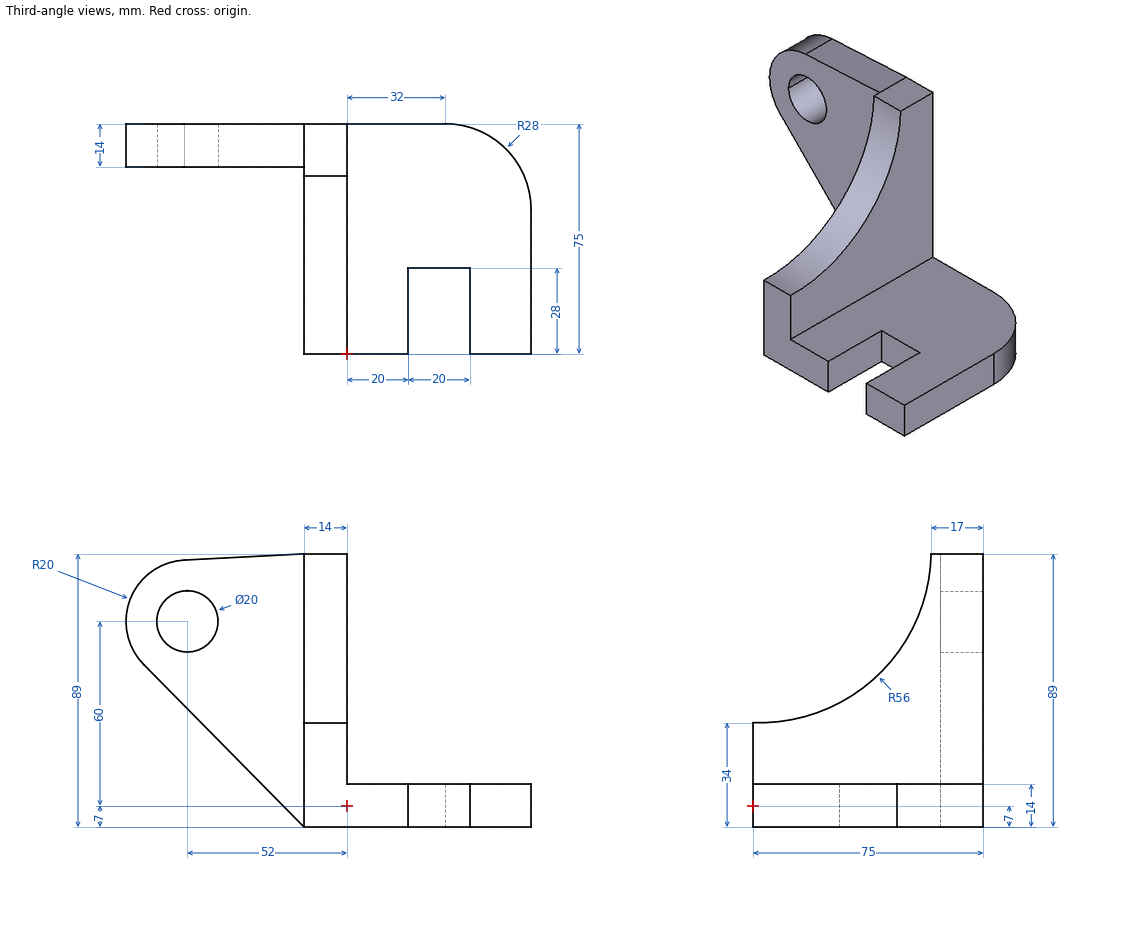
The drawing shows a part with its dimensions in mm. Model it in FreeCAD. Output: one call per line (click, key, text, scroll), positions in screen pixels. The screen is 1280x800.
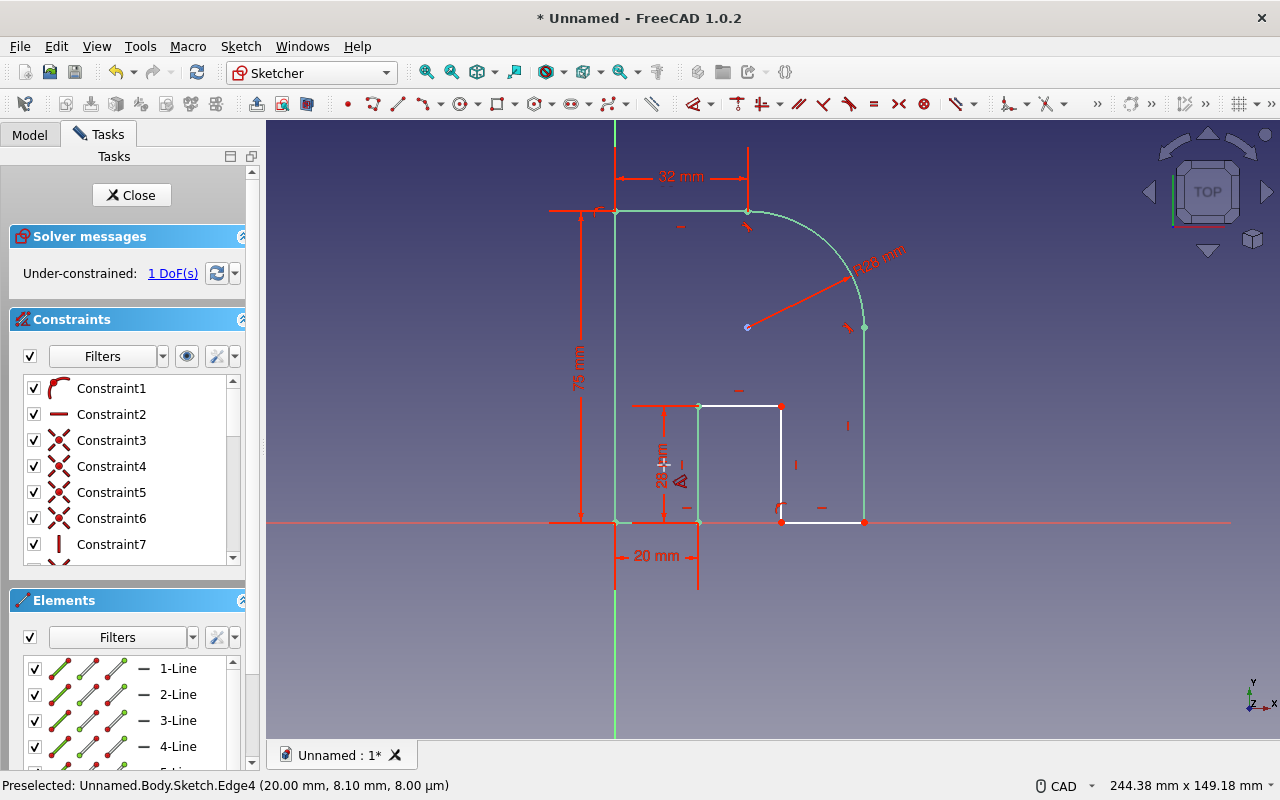
click(723, 406)
click(740, 440)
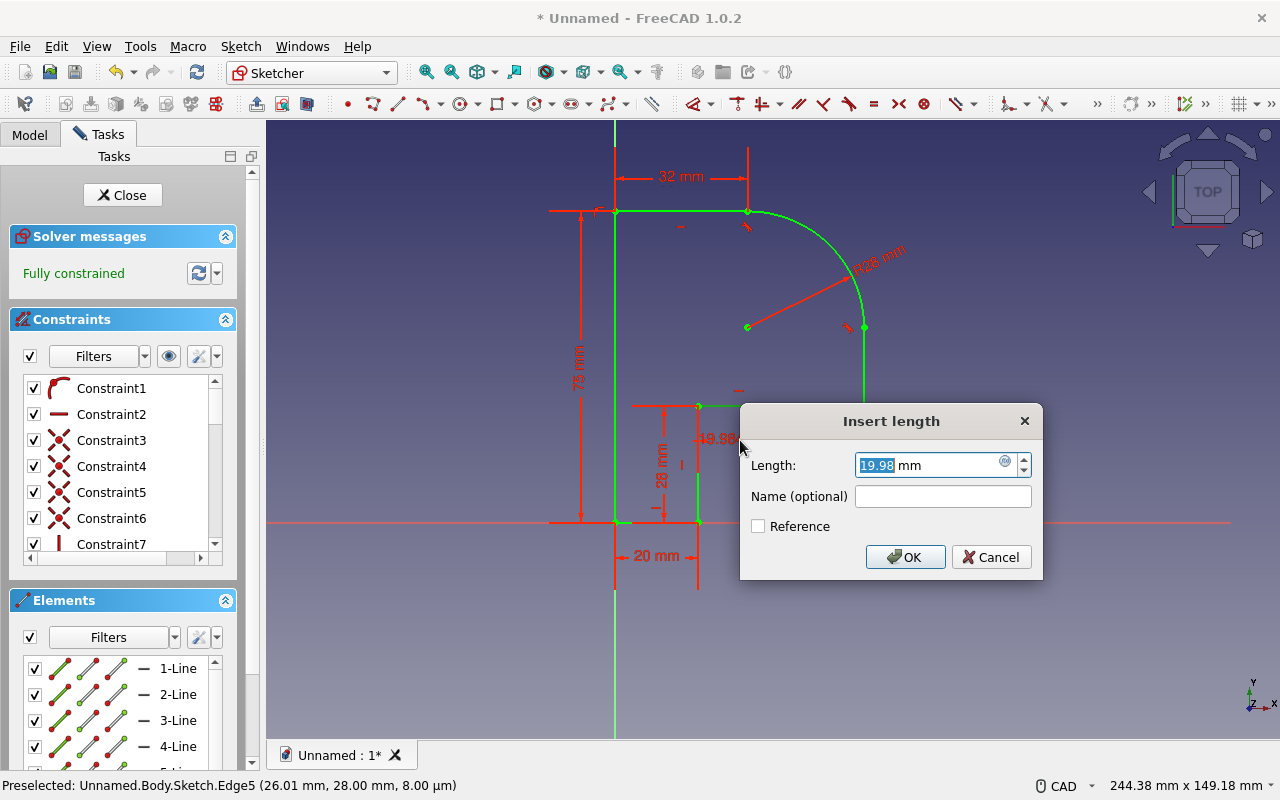
text(20)
key(Return)
key(Escape)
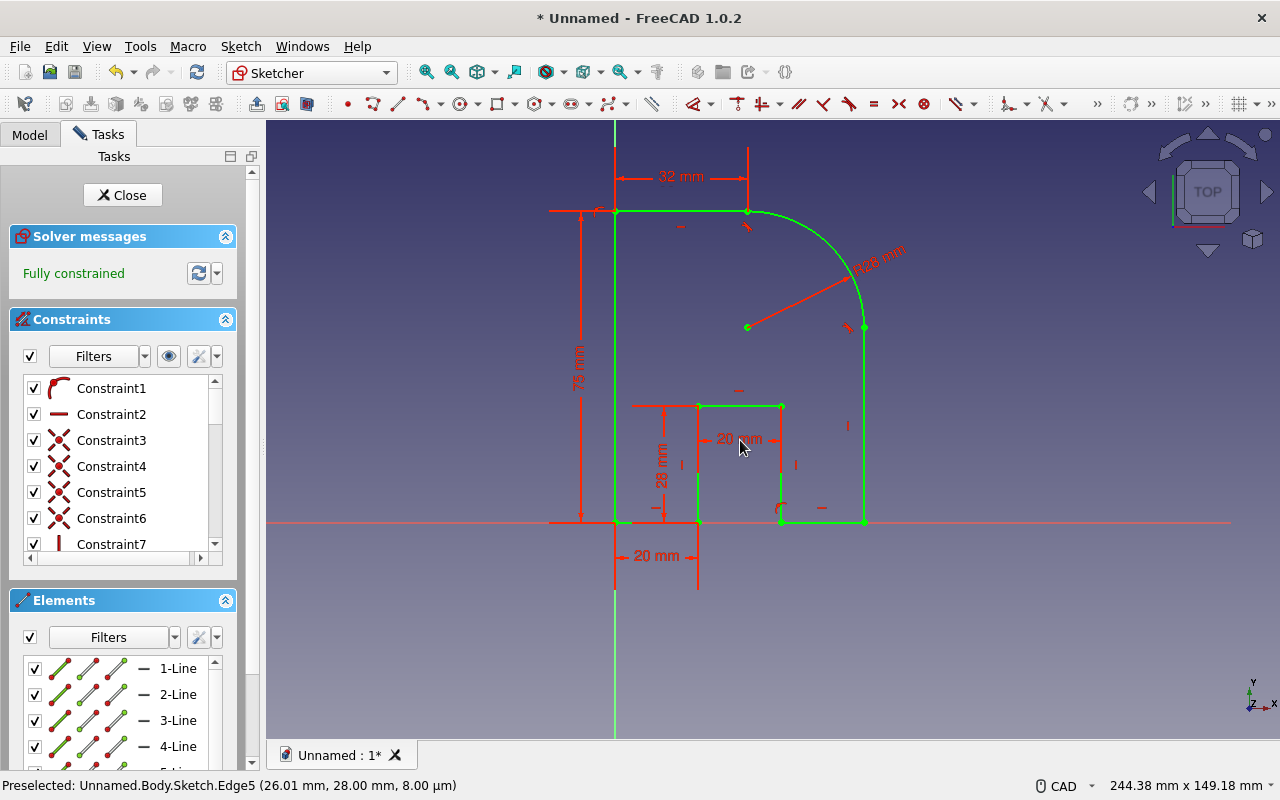
click(123, 195)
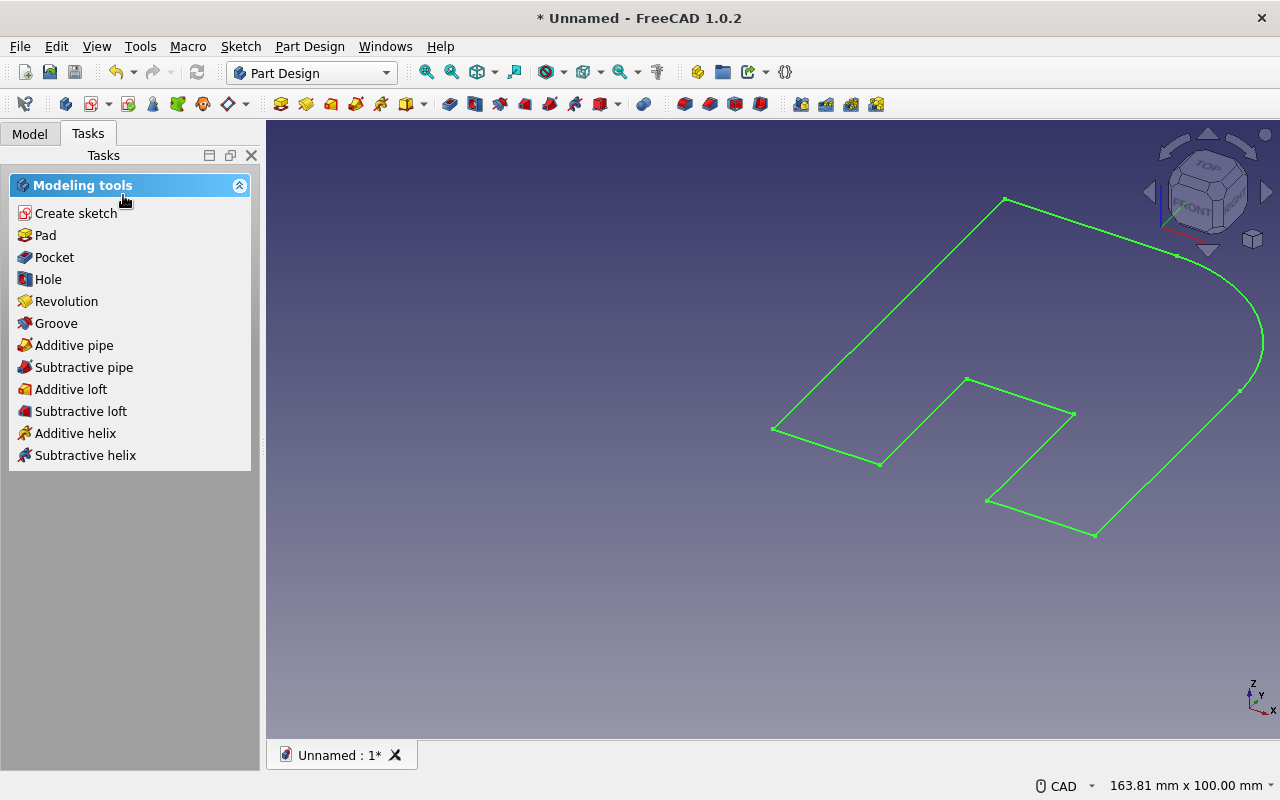
click(281, 104)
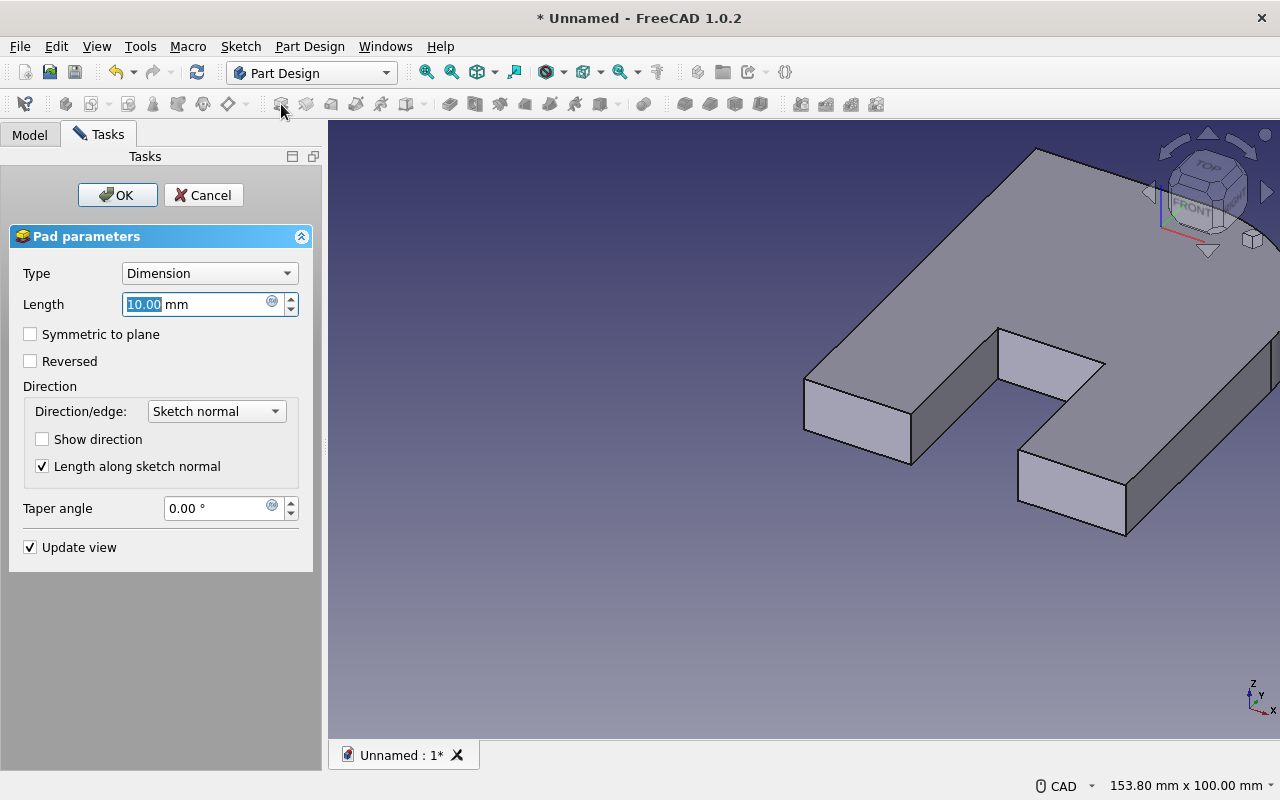
text(14)
key(Tab)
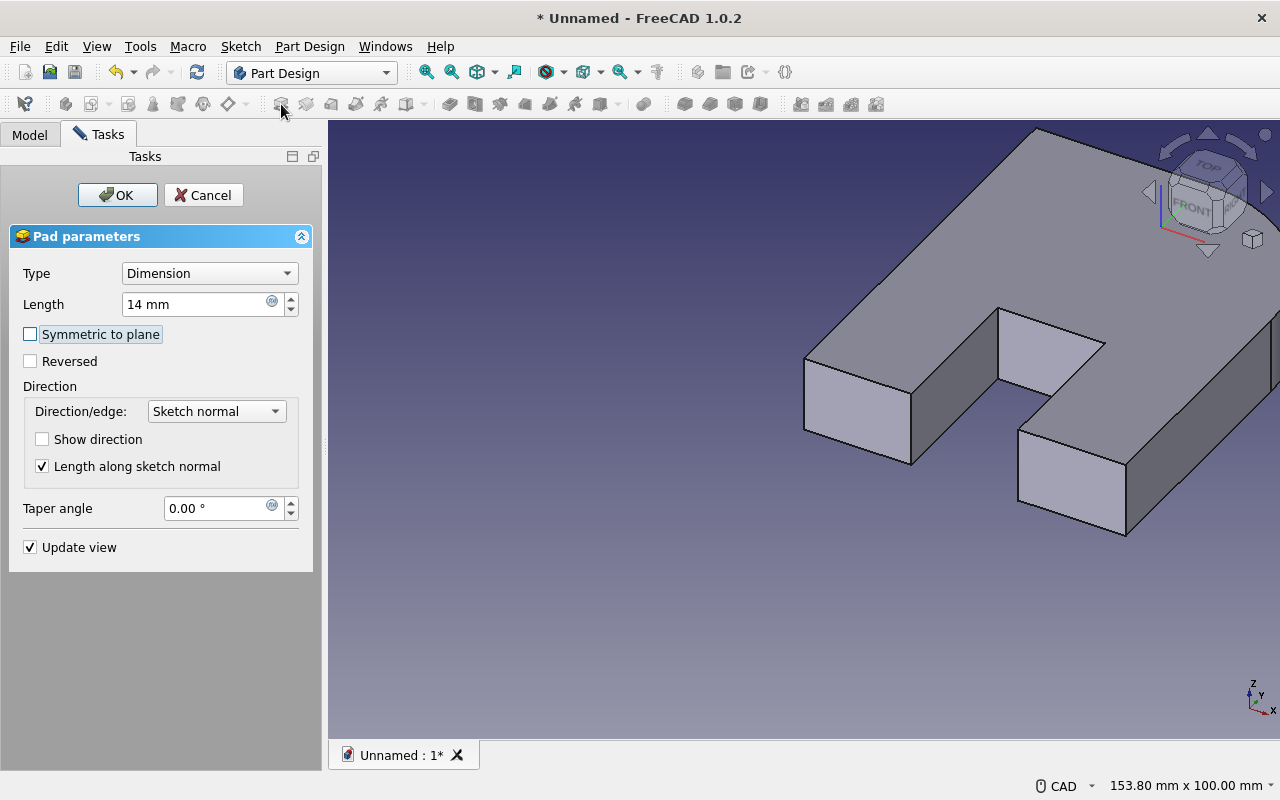
click(31, 334)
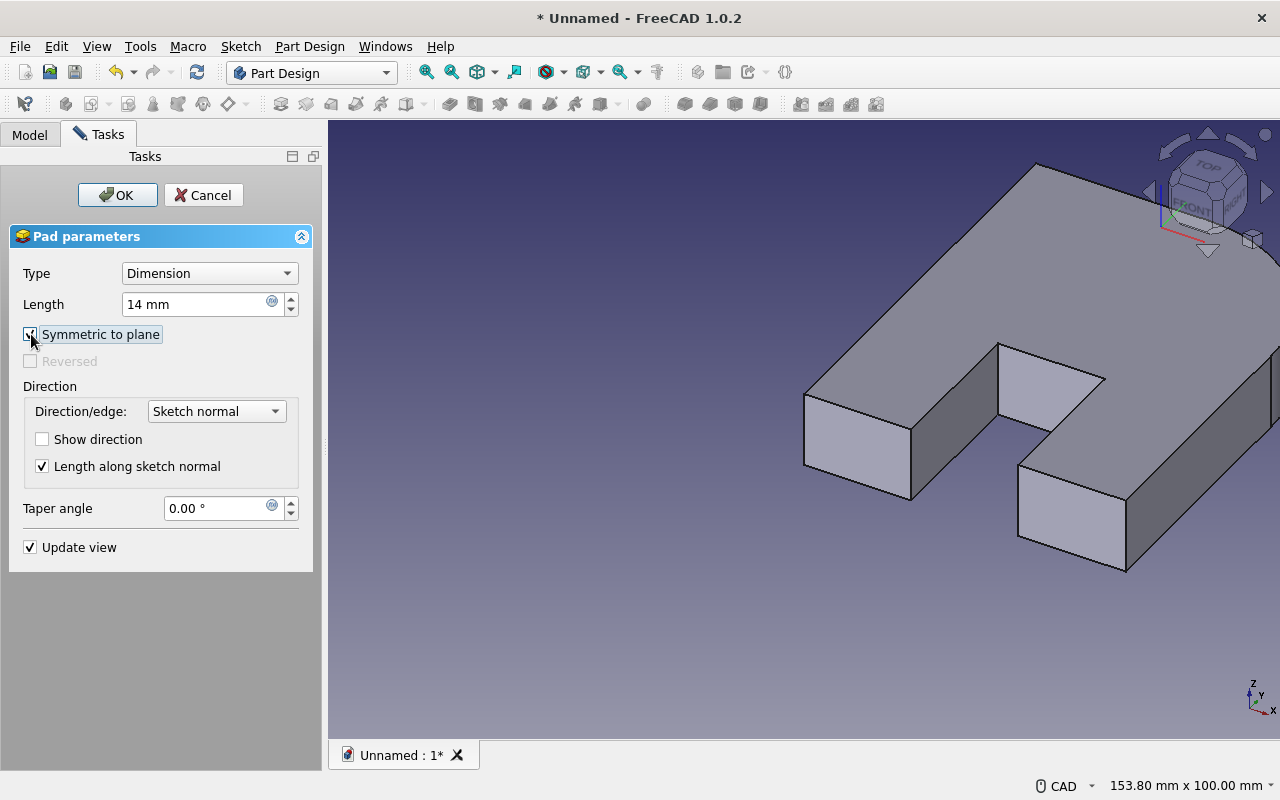
click(118, 195)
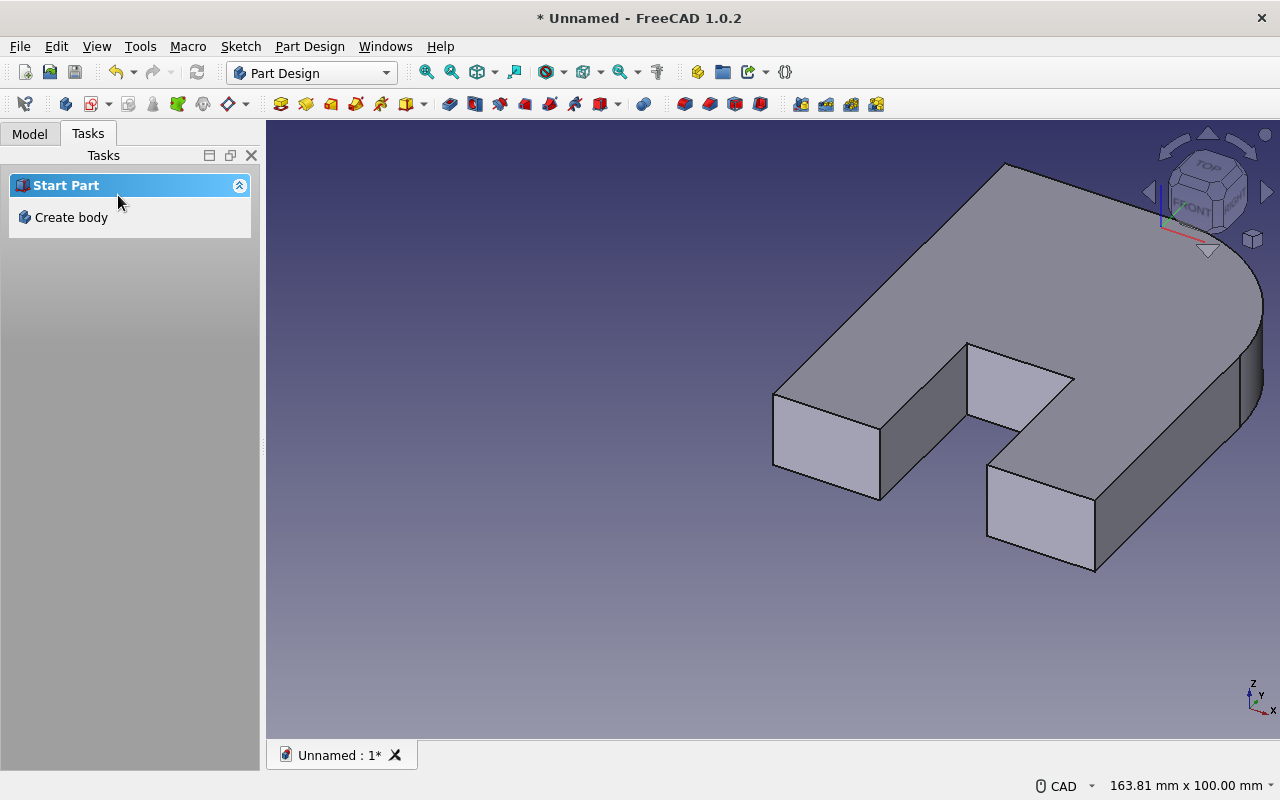
click(427, 72)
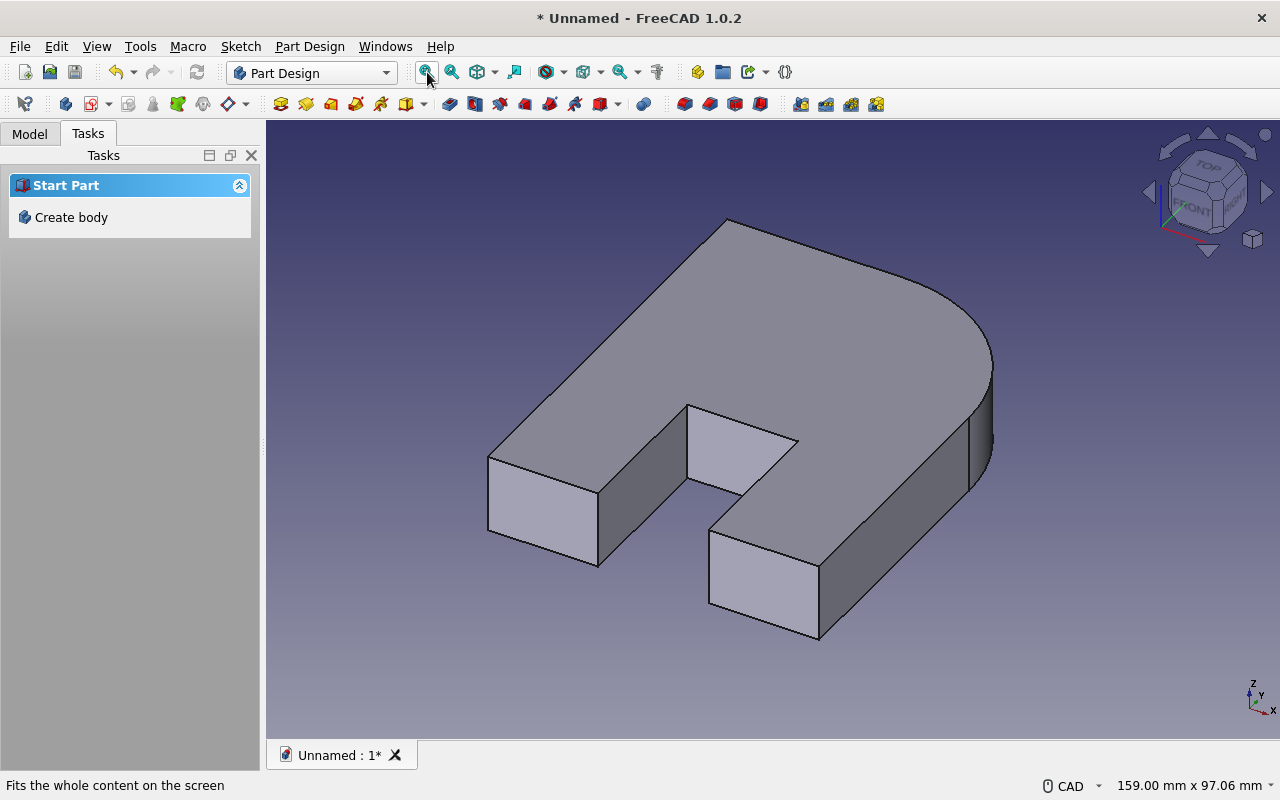
key(6)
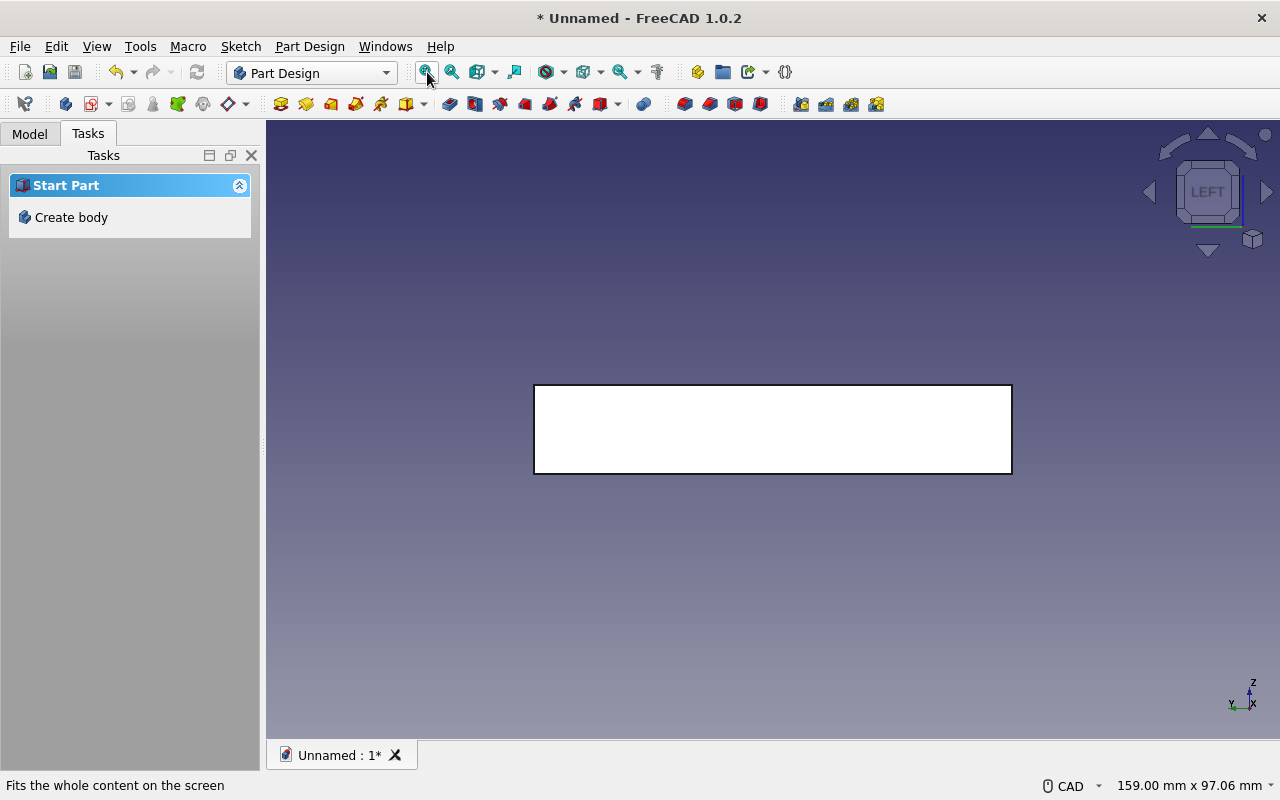
click(636, 428)